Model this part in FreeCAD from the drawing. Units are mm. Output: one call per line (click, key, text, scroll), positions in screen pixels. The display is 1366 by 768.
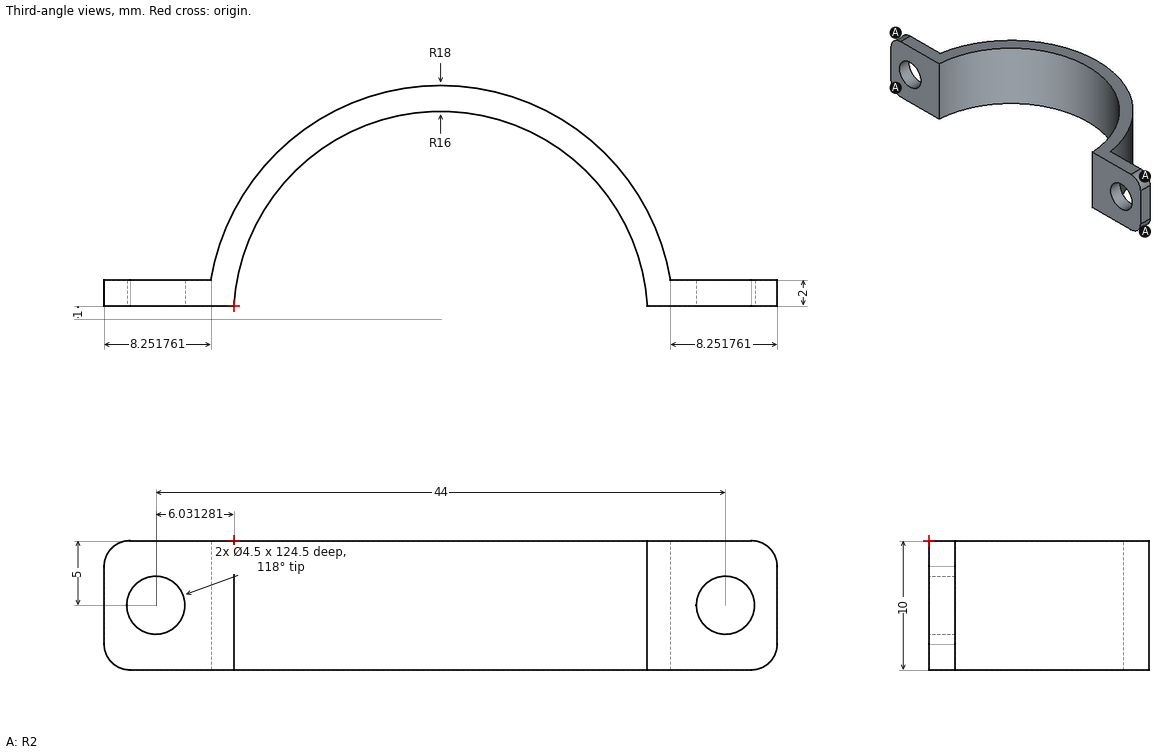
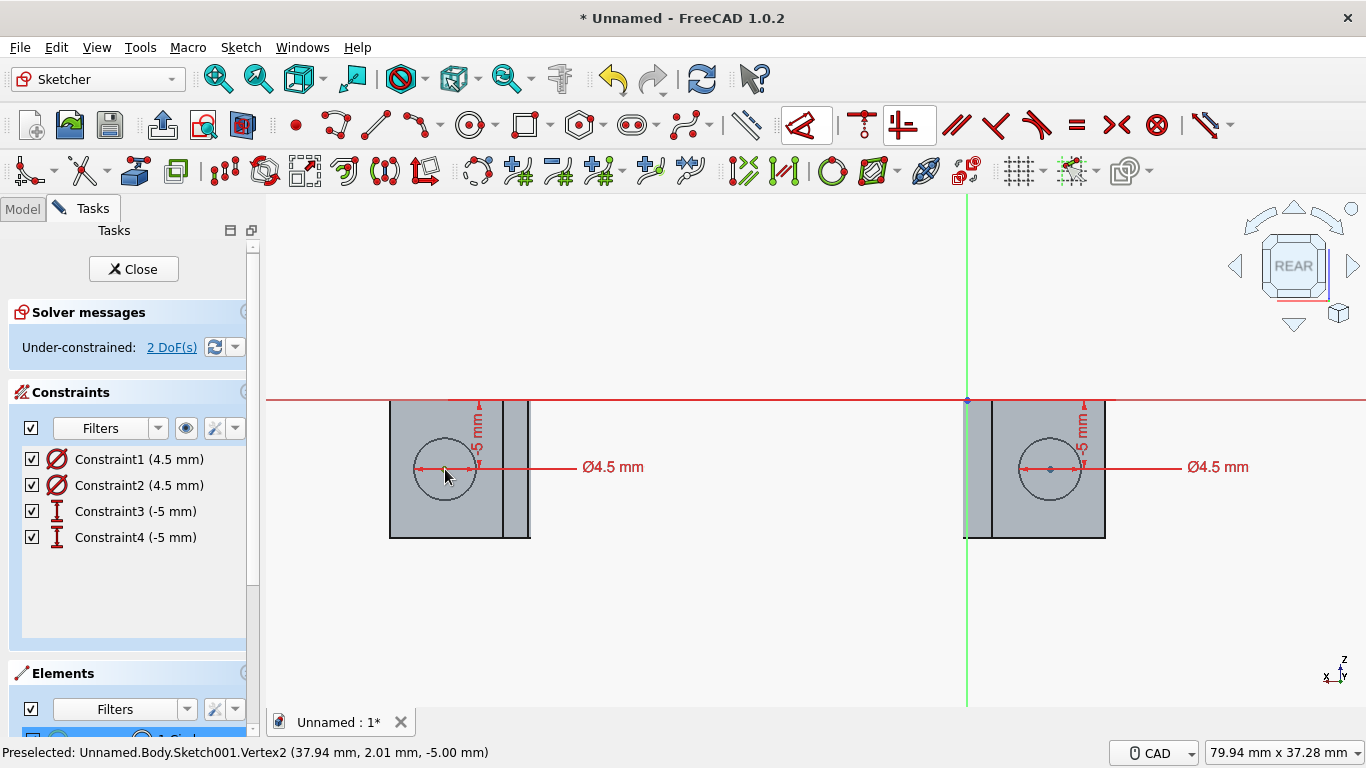
click(826, 126)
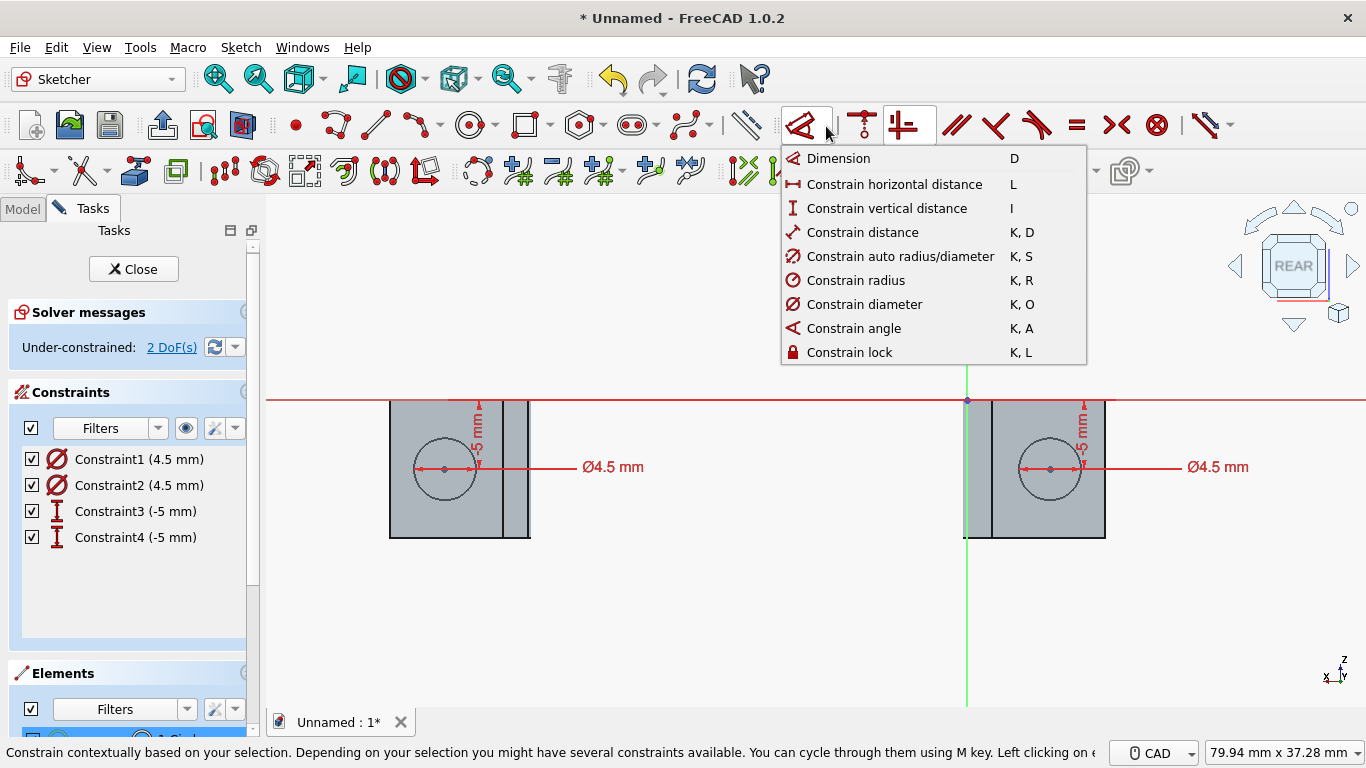
click(934, 184)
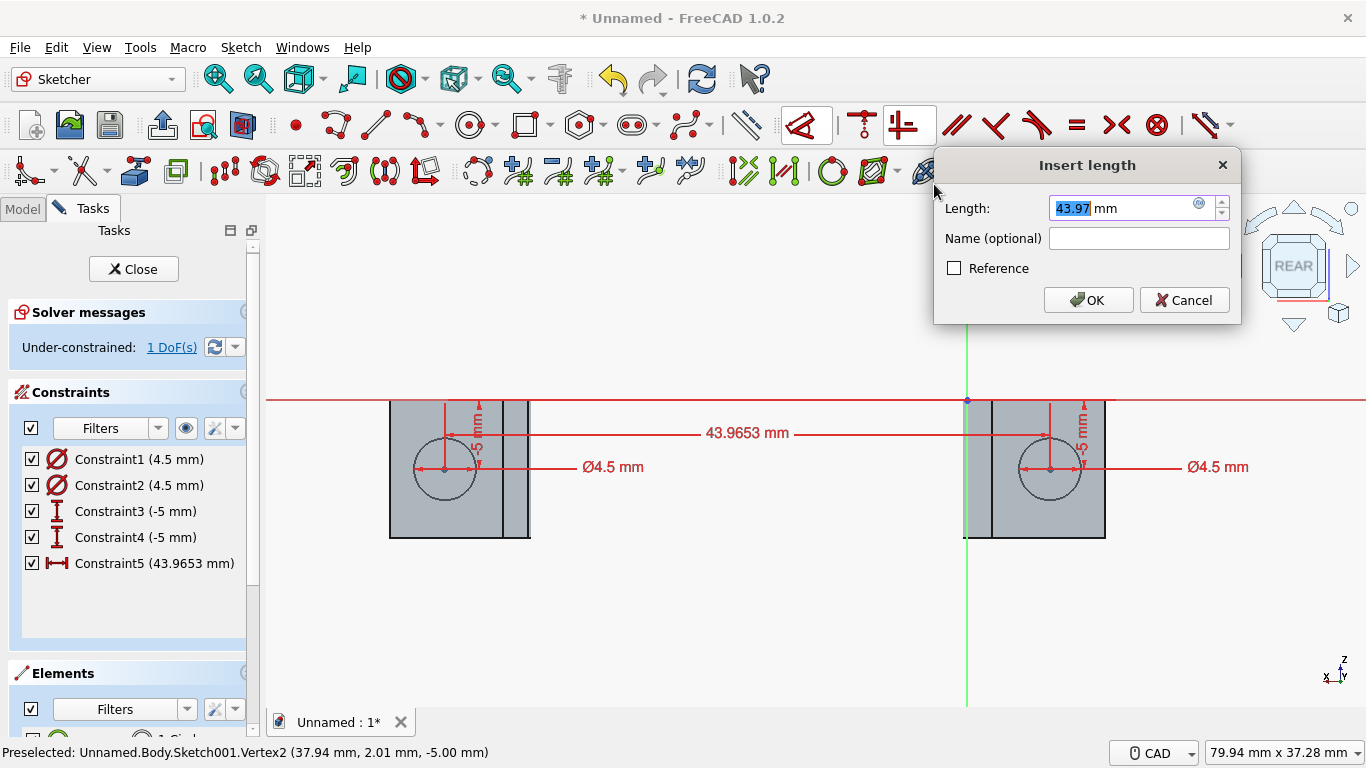
text(44)
key(Return)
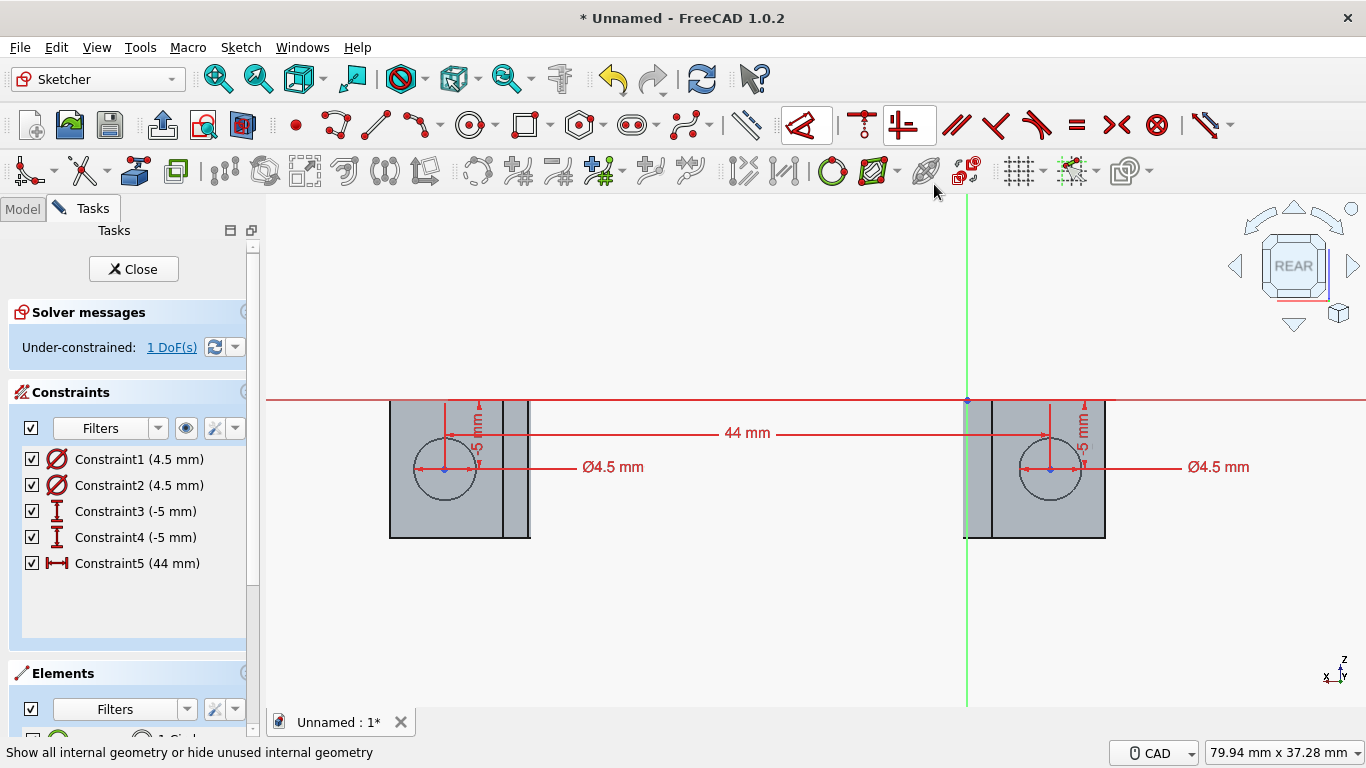
click(1050, 469)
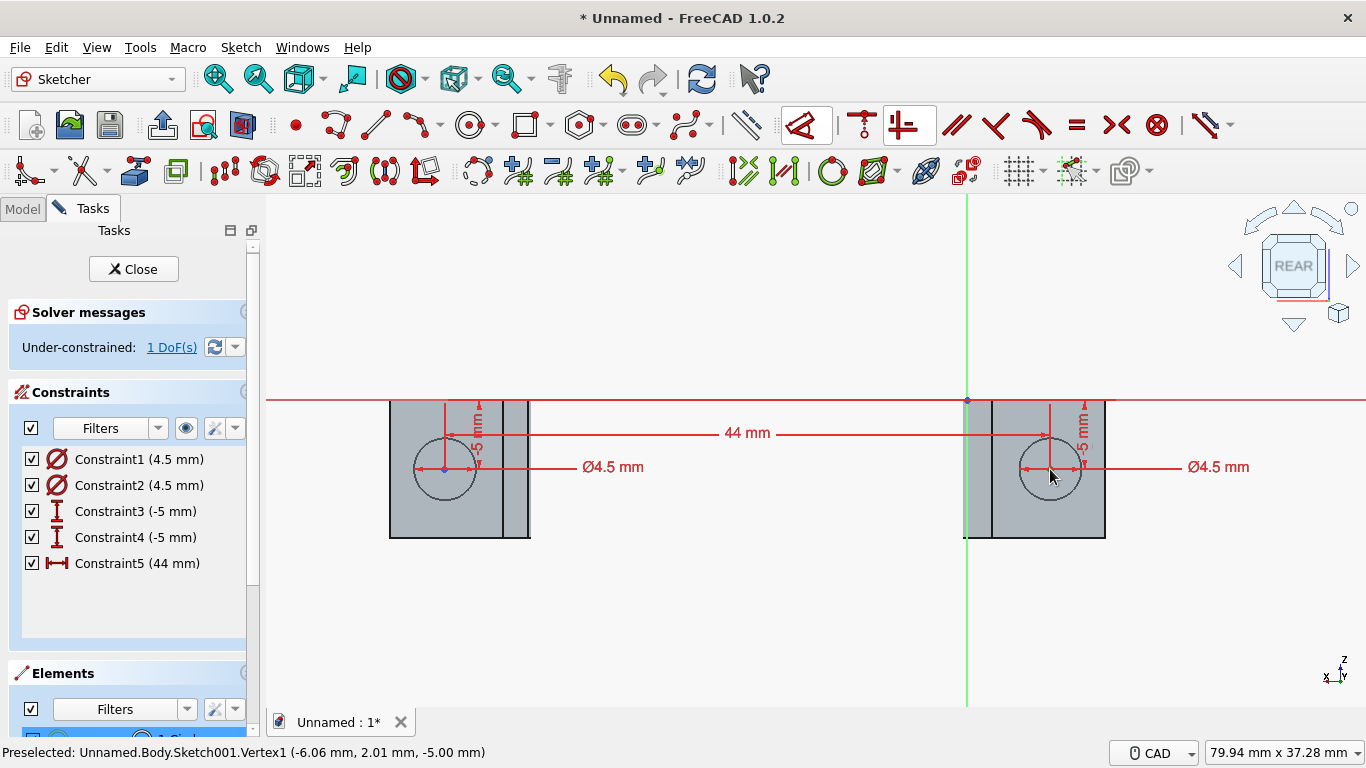
key(l)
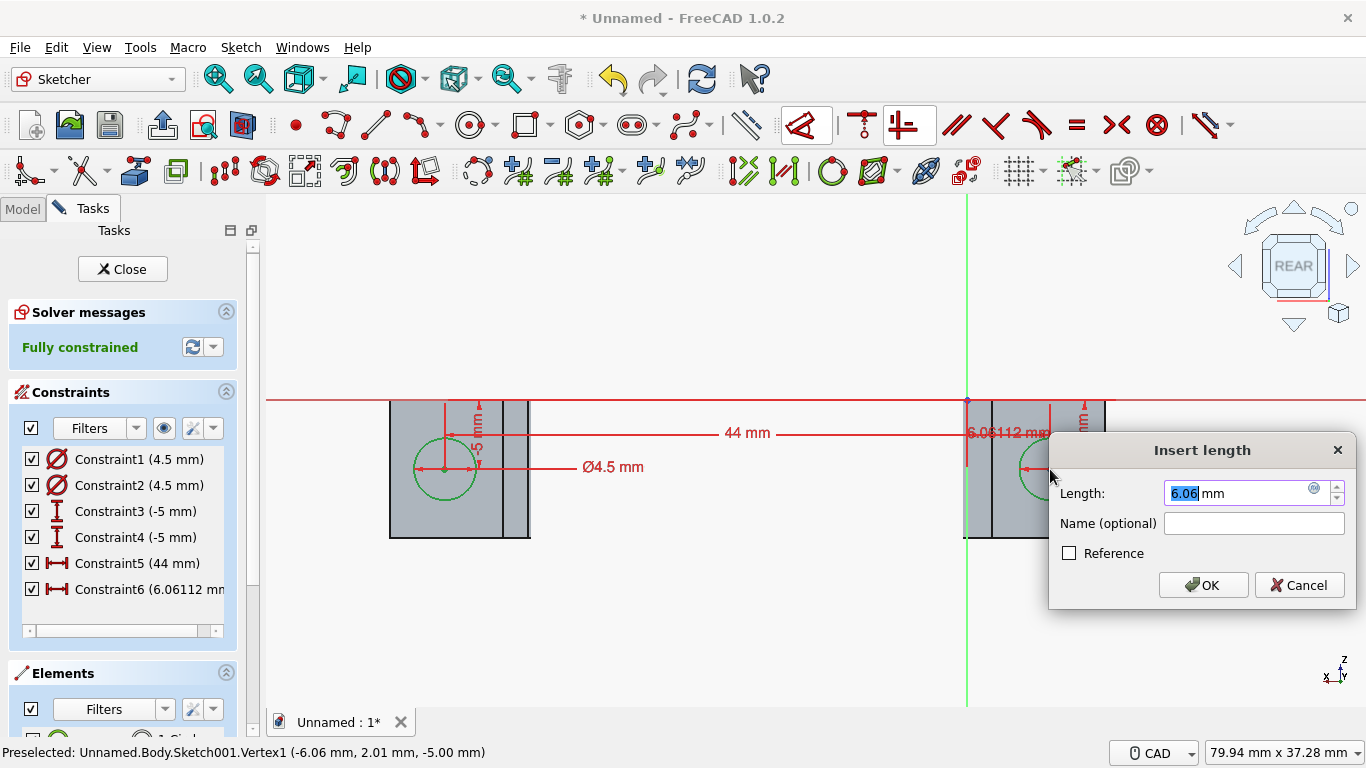
text(6.031281)
key(Return)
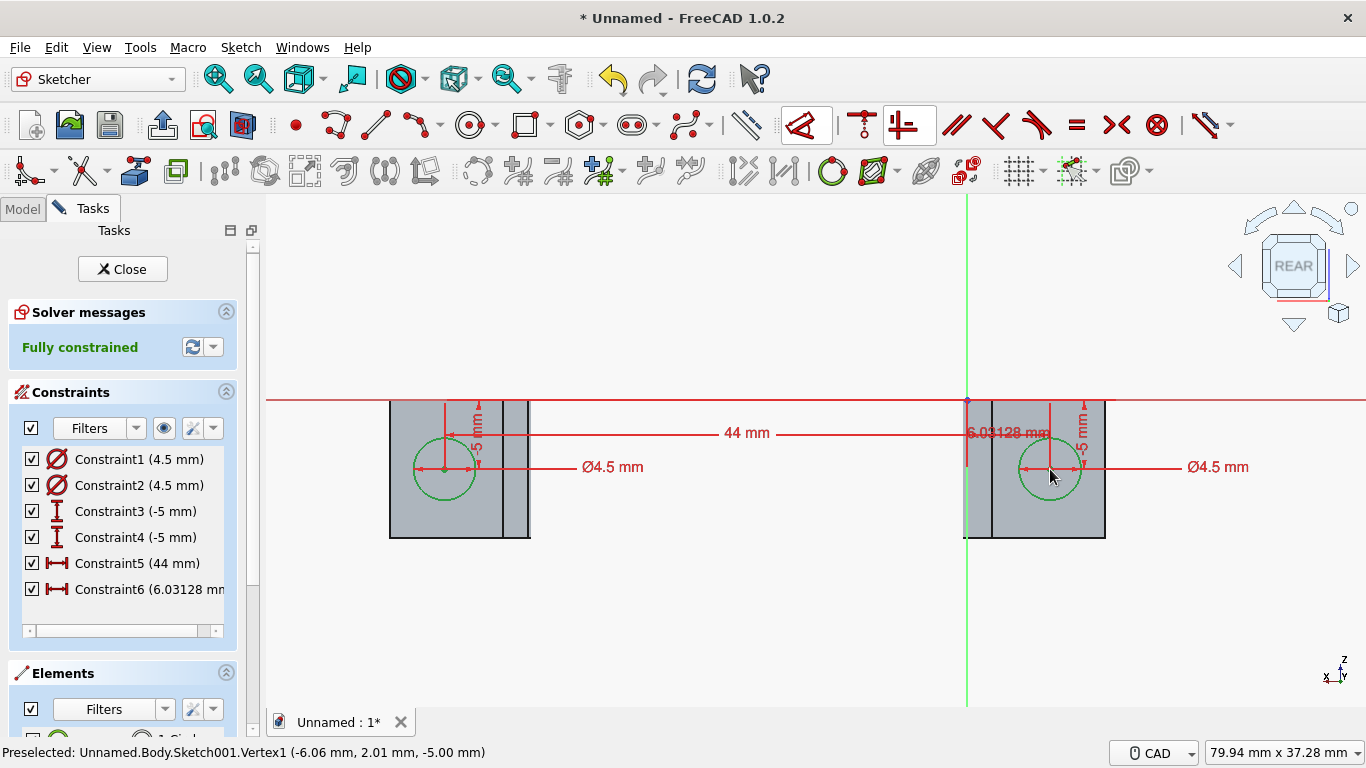
click(123, 269)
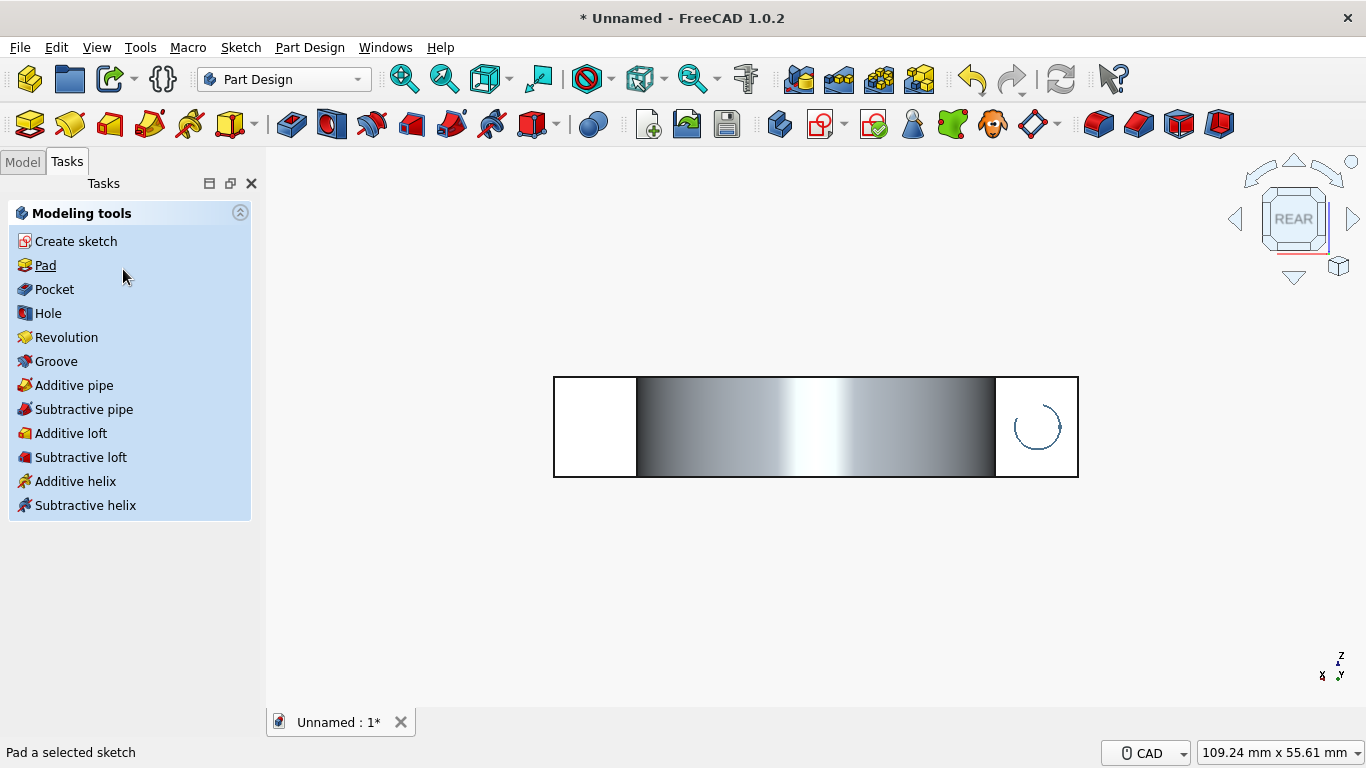
click(332, 124)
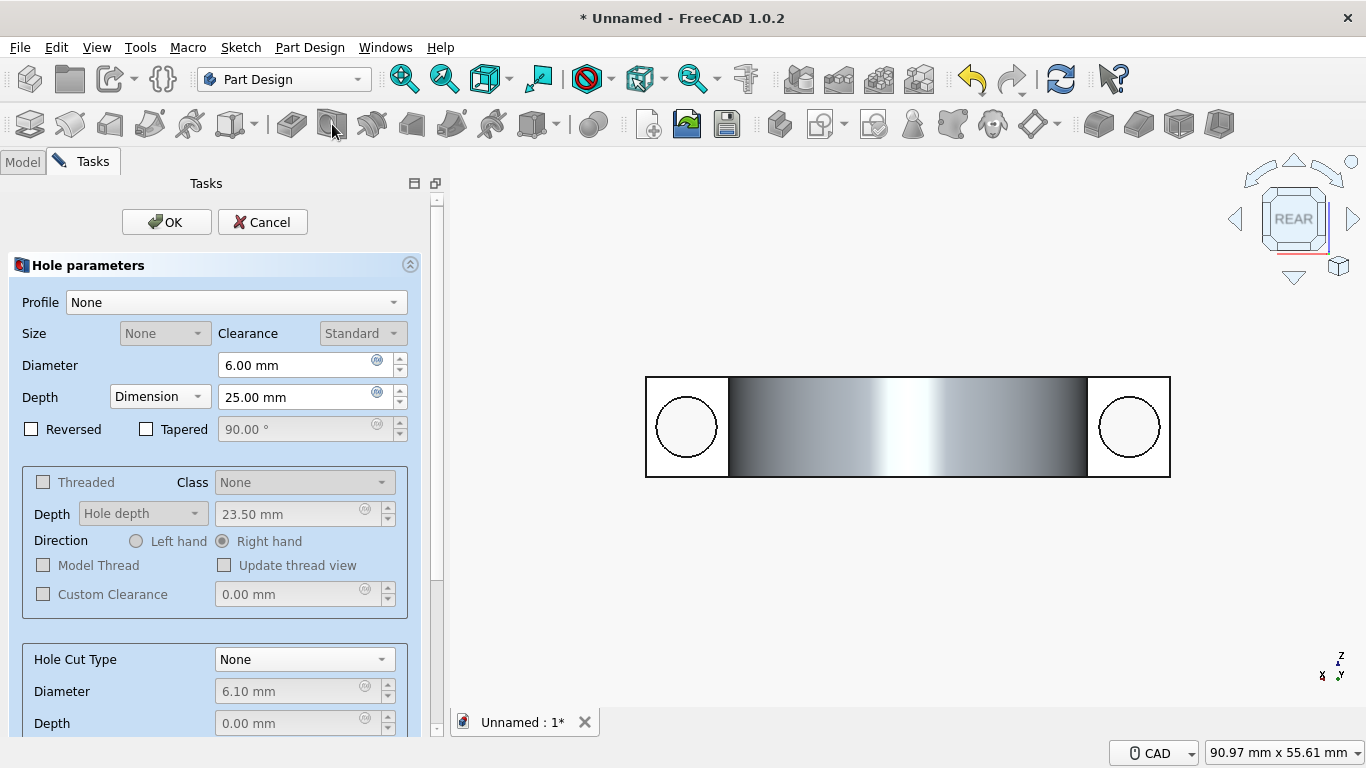
triple_click(305, 365)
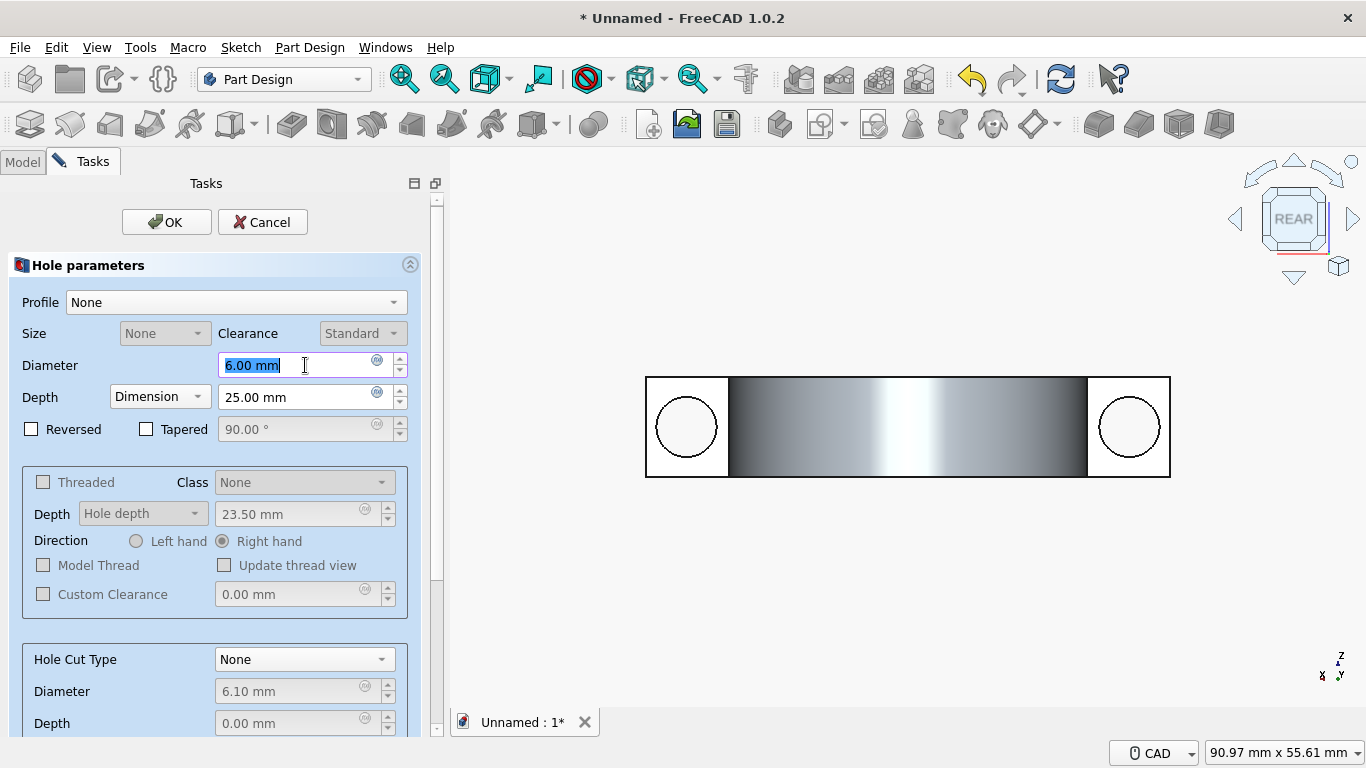
text(4.5)
key(Tab)